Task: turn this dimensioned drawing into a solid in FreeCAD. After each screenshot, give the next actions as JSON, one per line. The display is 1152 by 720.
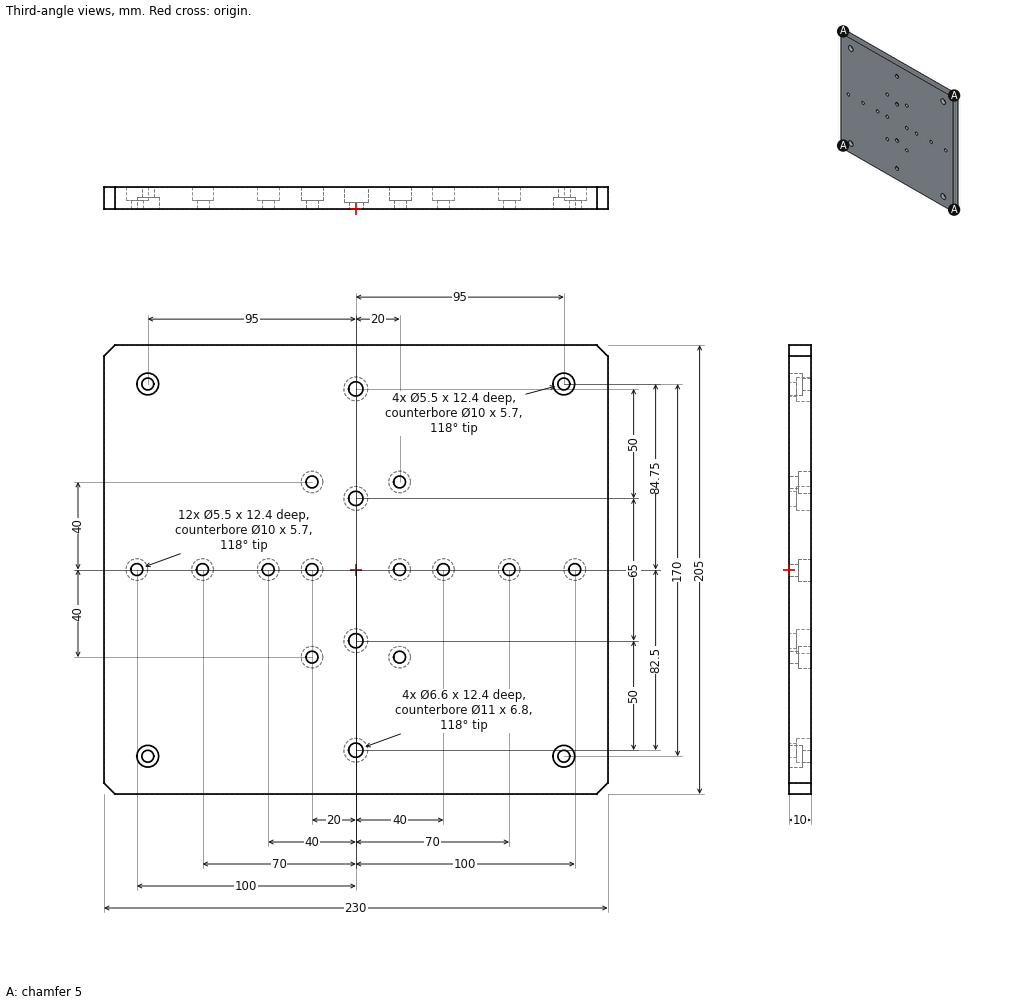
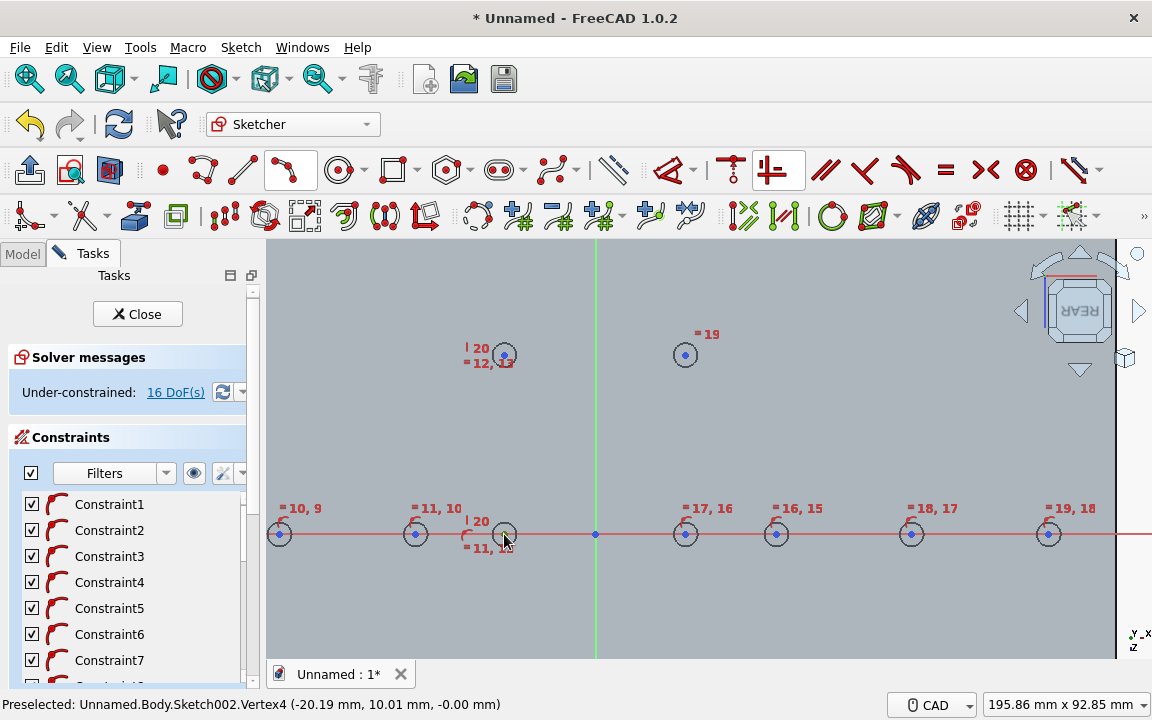
{"action": "scroll", "coordinate": [695, 345], "scroll_direction": "down", "scroll_amount": 3}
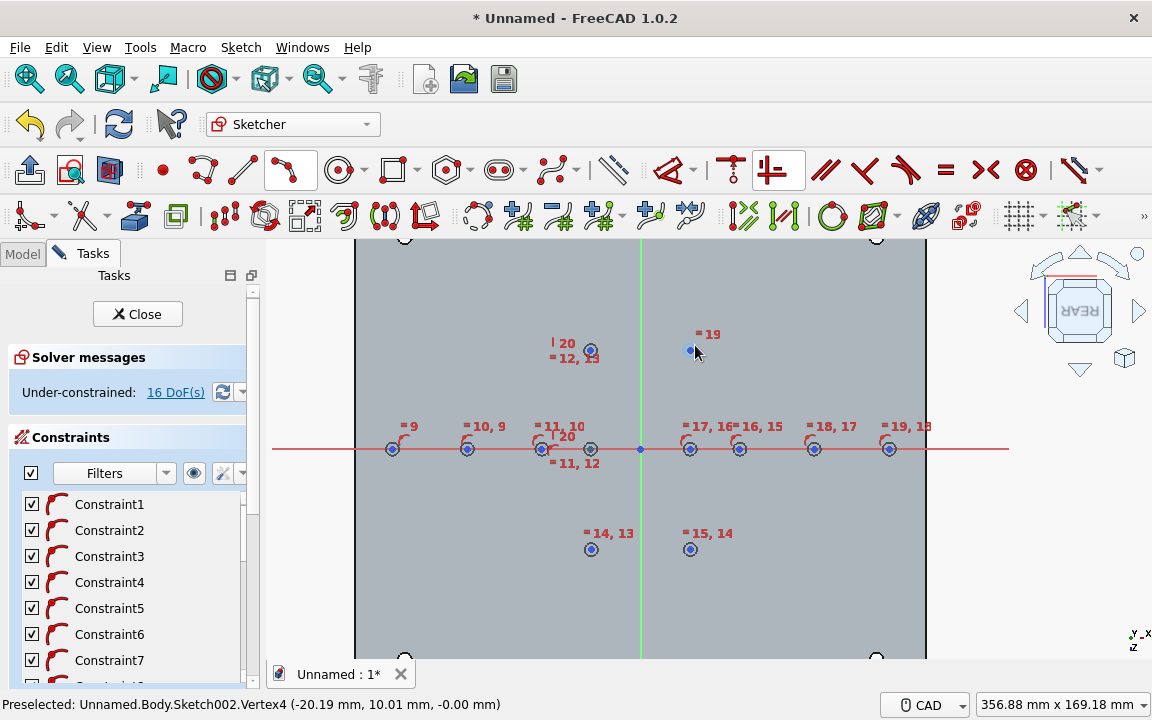
{"action": "left_click", "coordinate": [591, 550]}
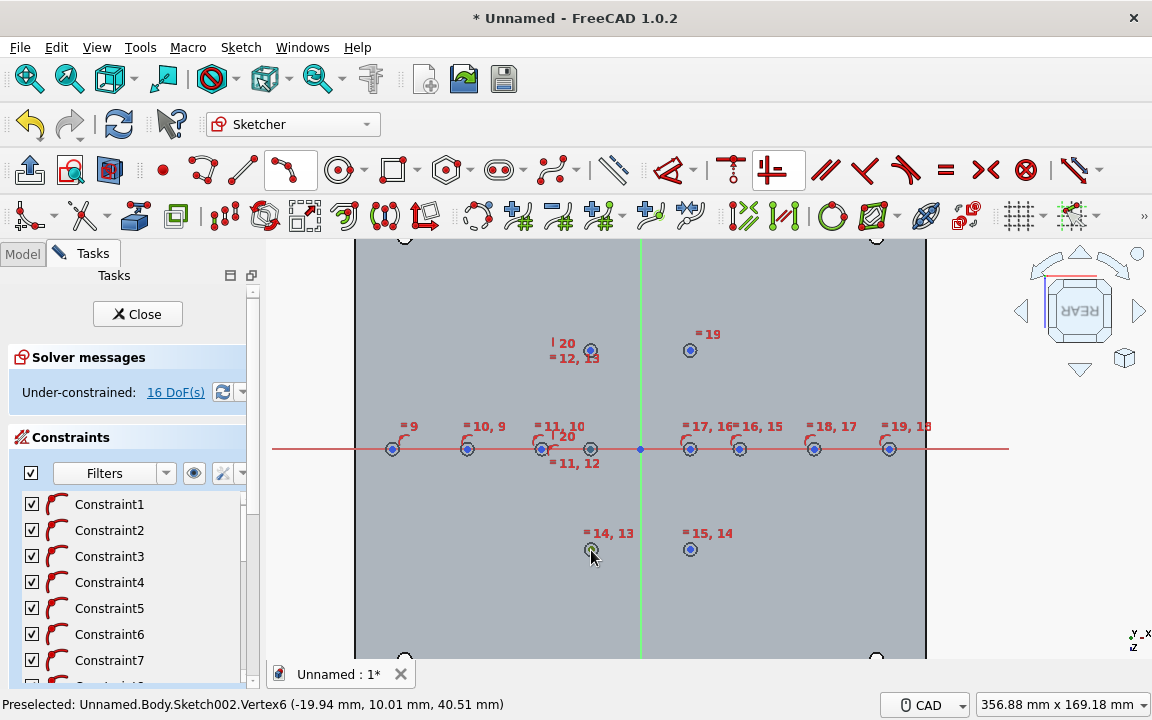
{"action": "left_click", "coordinate": [800, 170]}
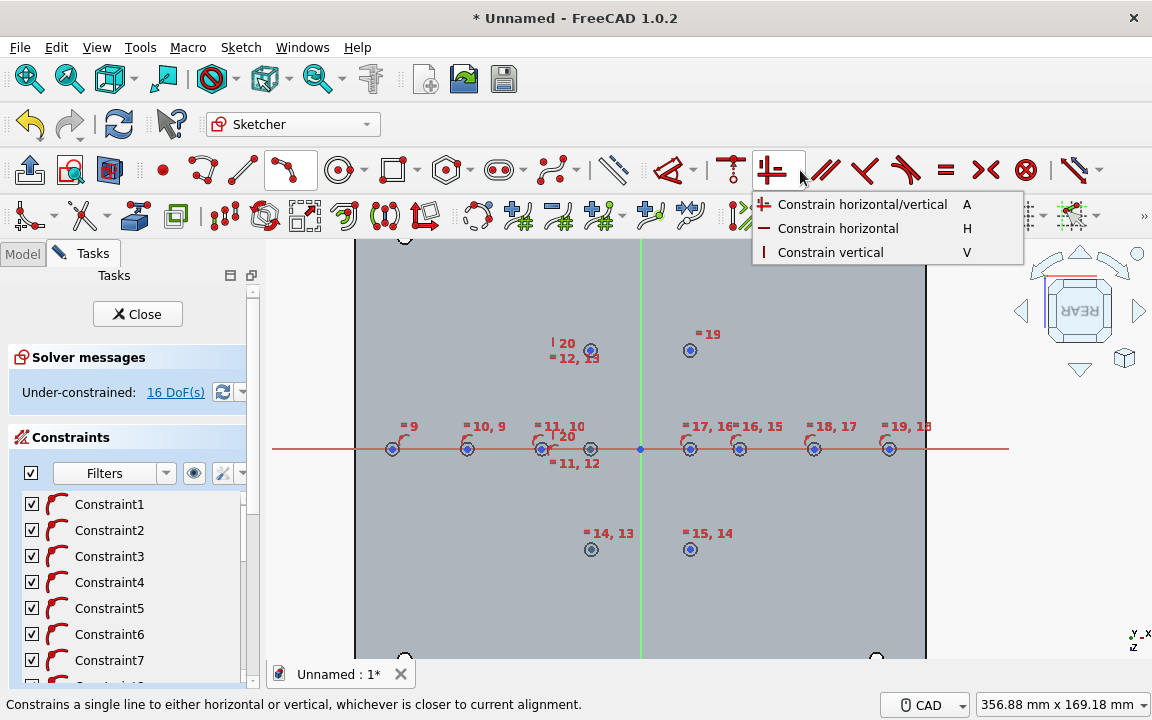
{"action": "left_click", "coordinate": [888, 252]}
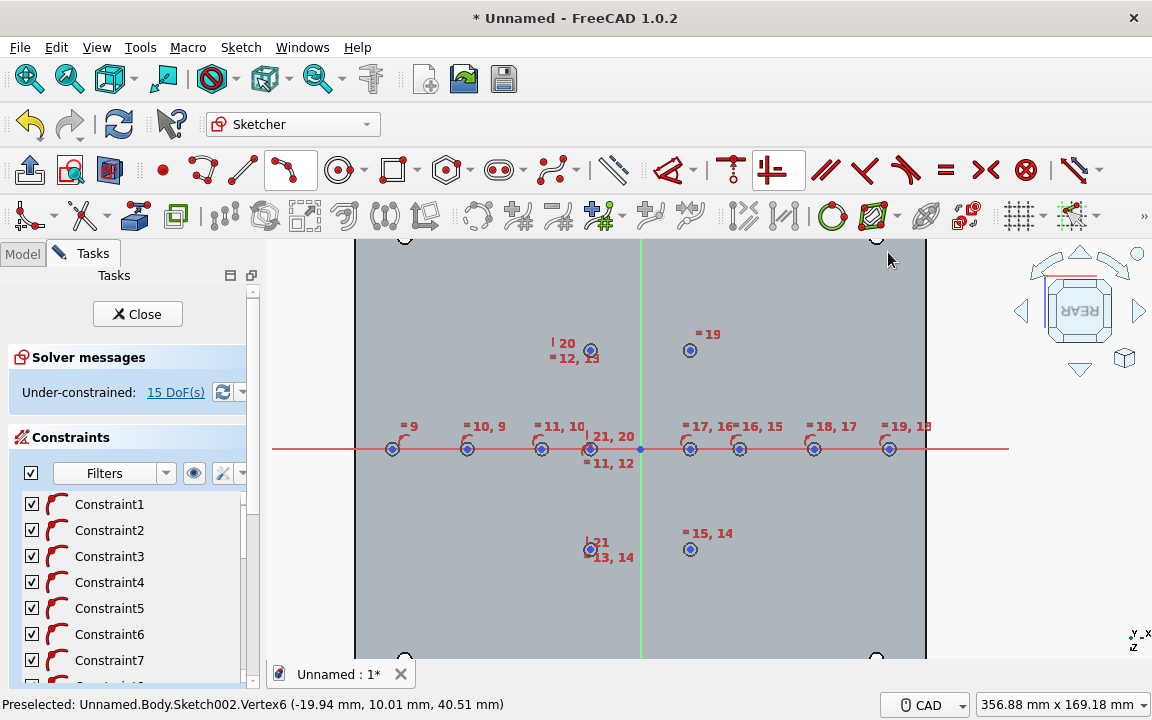
{"action": "scroll", "coordinate": [591, 550], "scroll_direction": "up", "scroll_amount": 4}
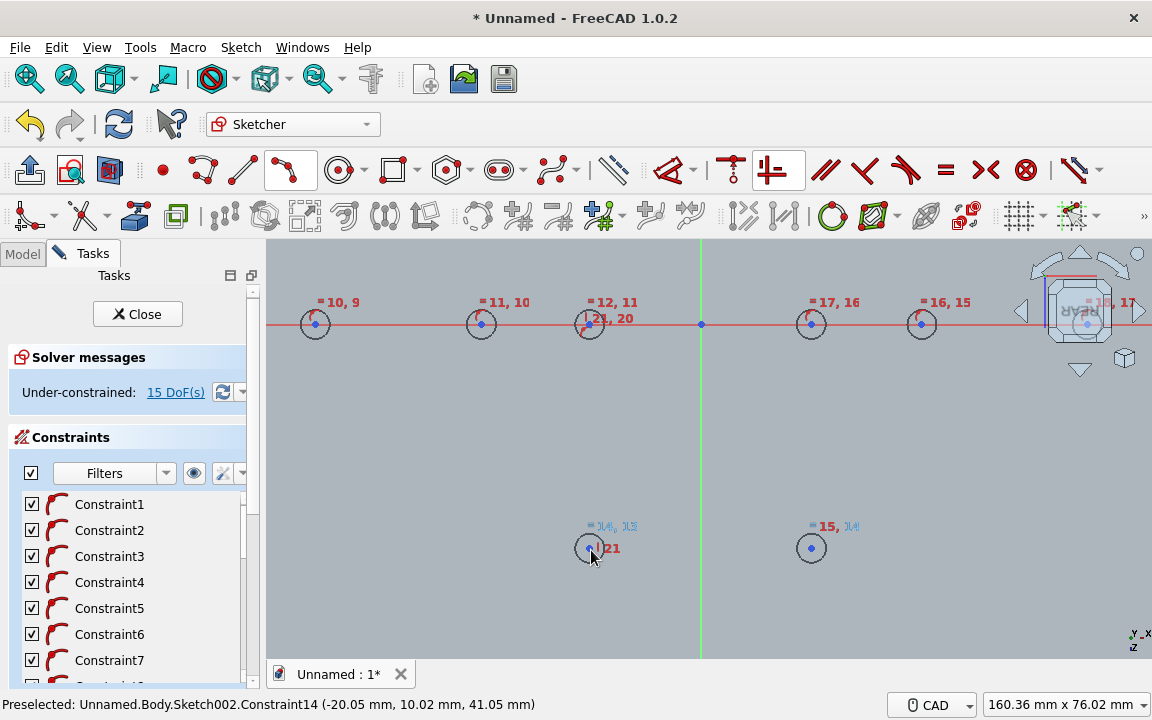
{"action": "left_click", "coordinate": [590, 548]}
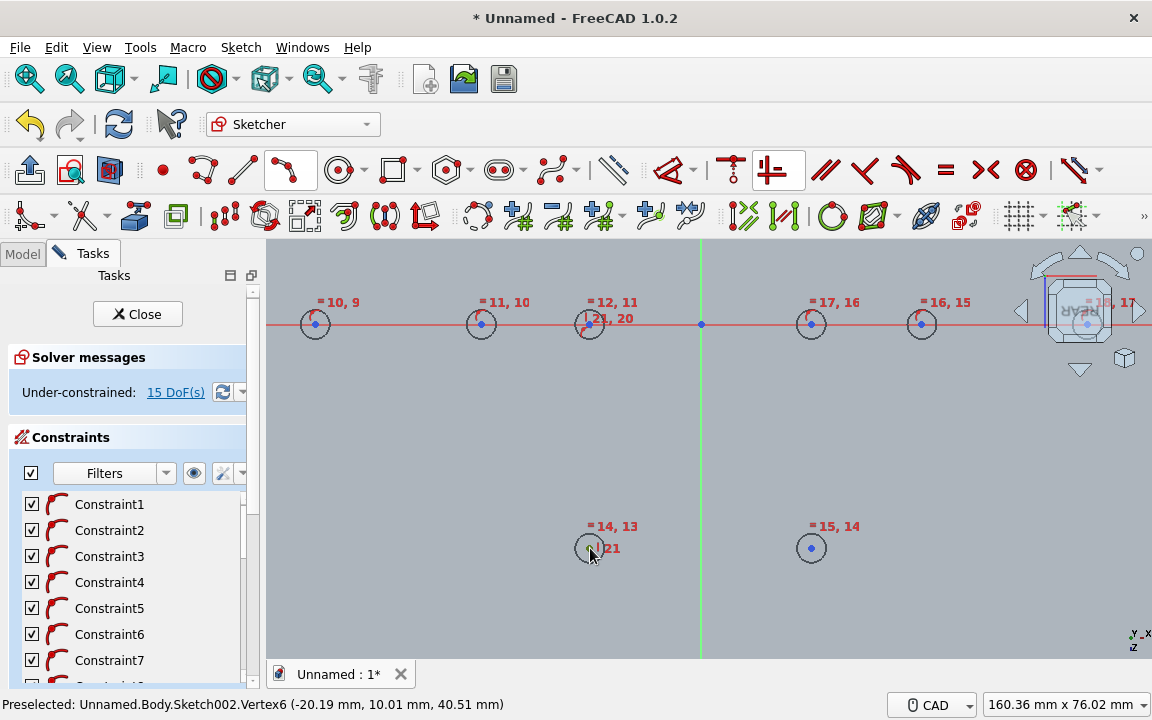
{"action": "left_click", "coordinate": [812, 548]}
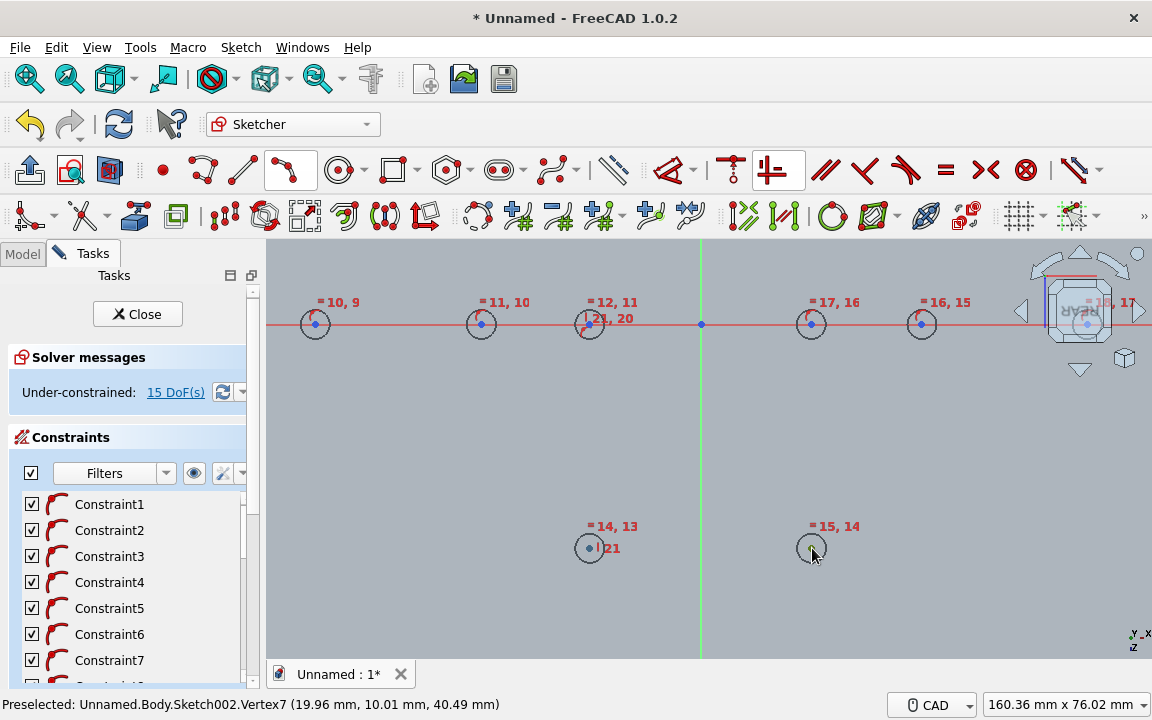
{"action": "left_click", "coordinate": [800, 170]}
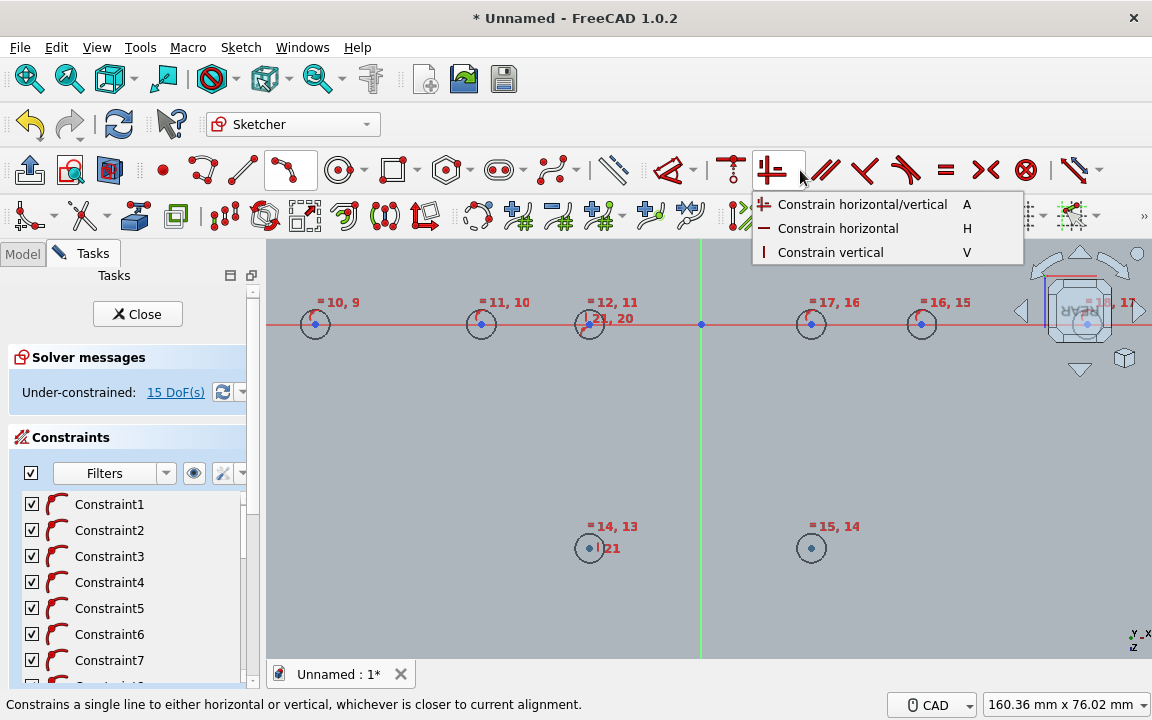
{"action": "left_click", "coordinate": [888, 228]}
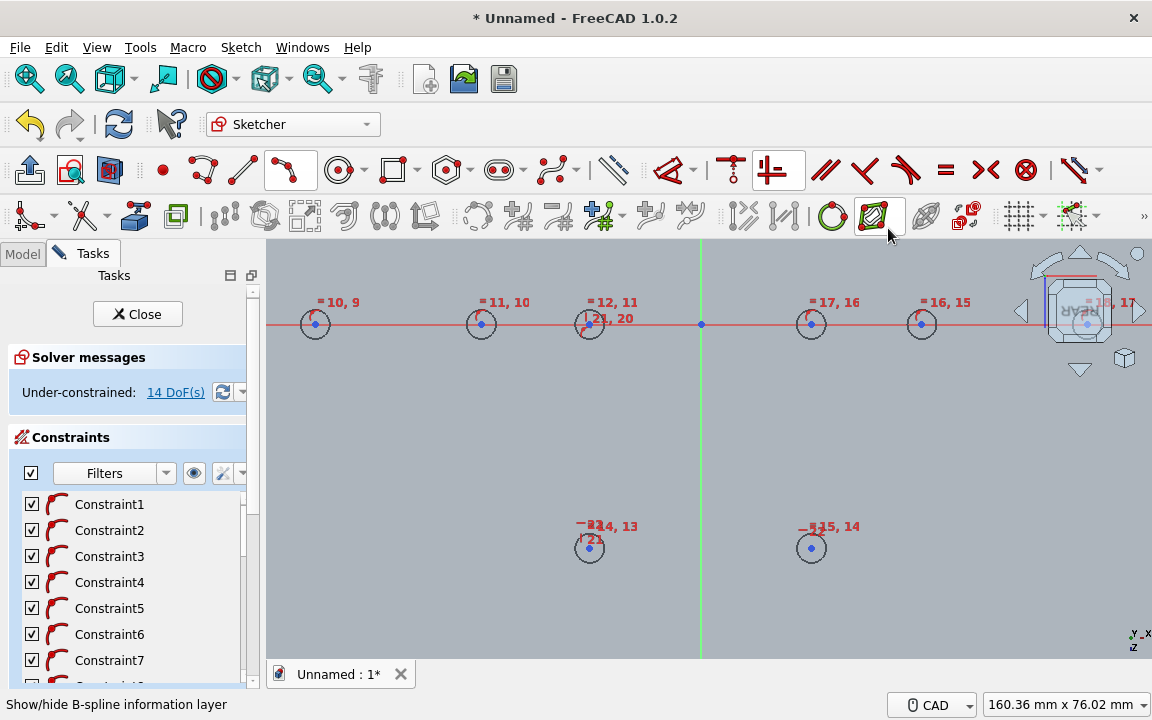
{"action": "left_click", "coordinate": [812, 548]}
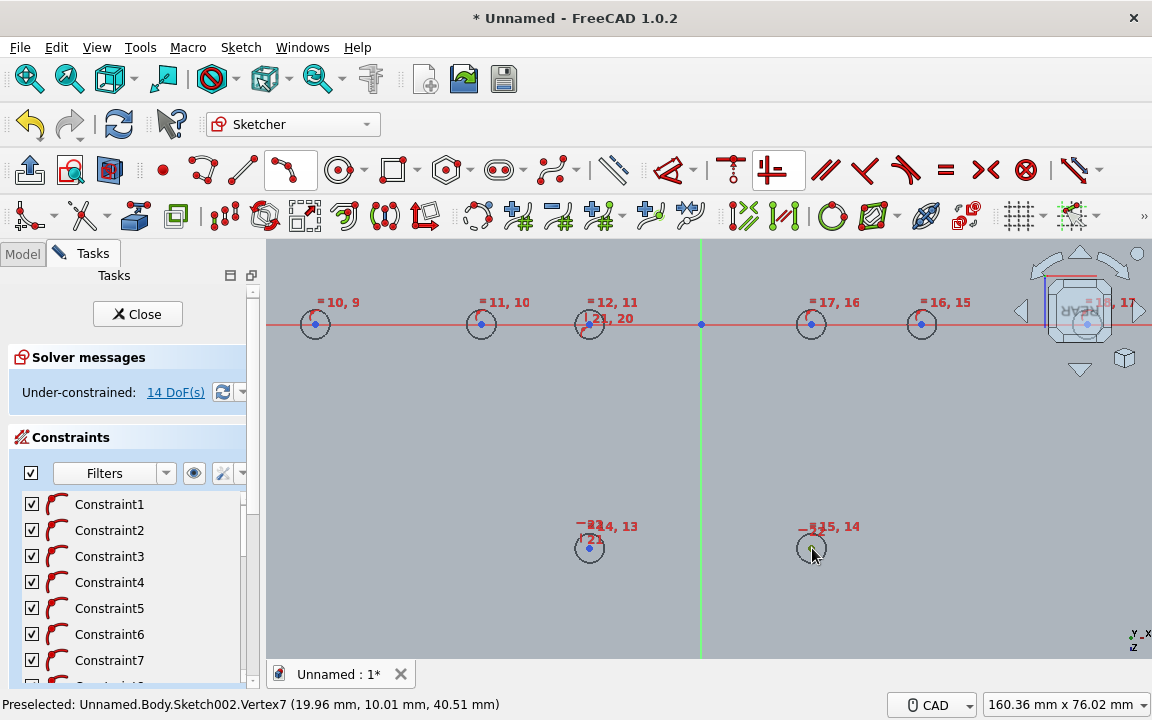
{"action": "left_click", "coordinate": [811, 325]}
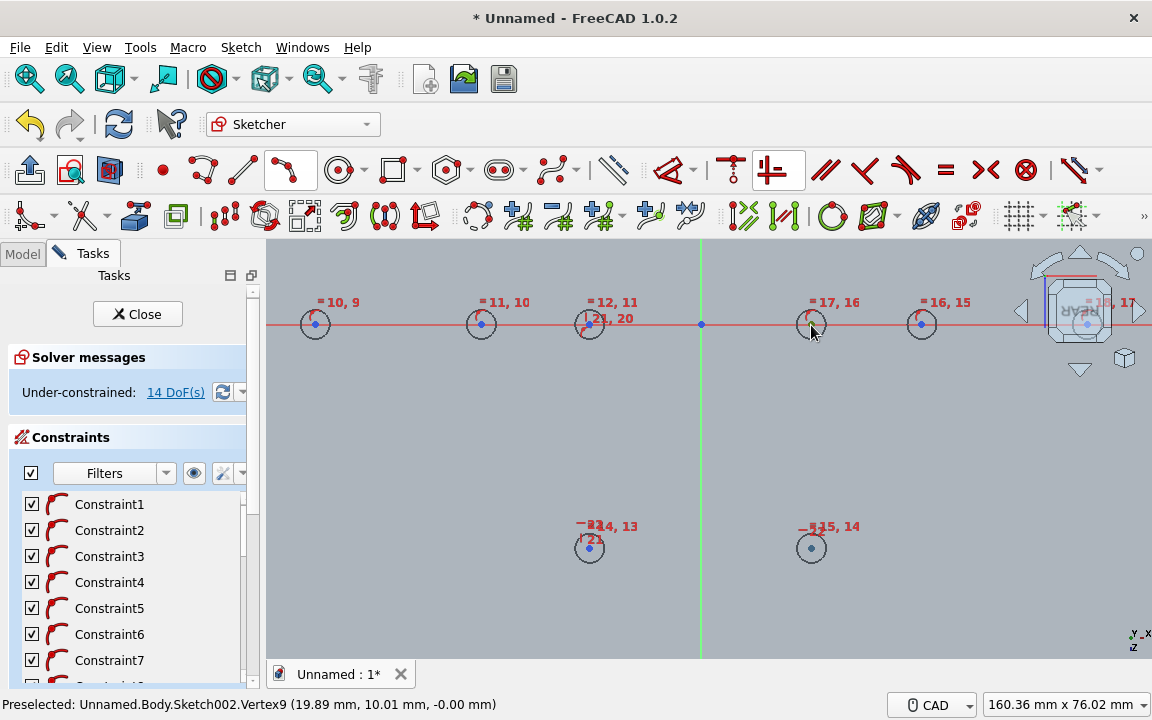
{"action": "left_click", "coordinate": [800, 170]}